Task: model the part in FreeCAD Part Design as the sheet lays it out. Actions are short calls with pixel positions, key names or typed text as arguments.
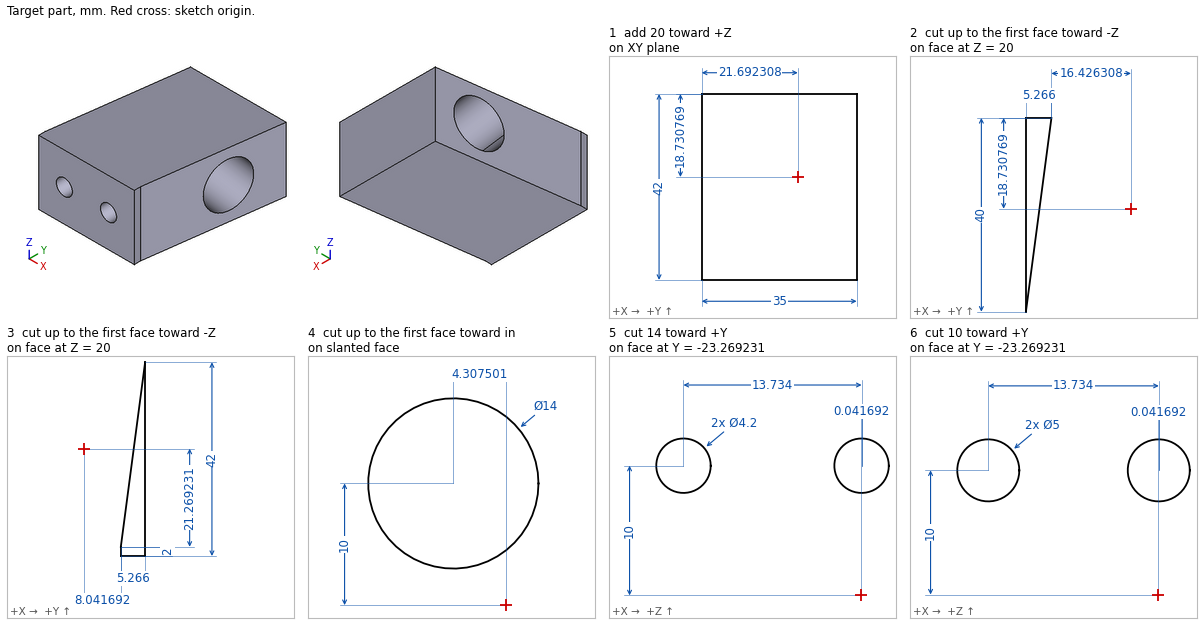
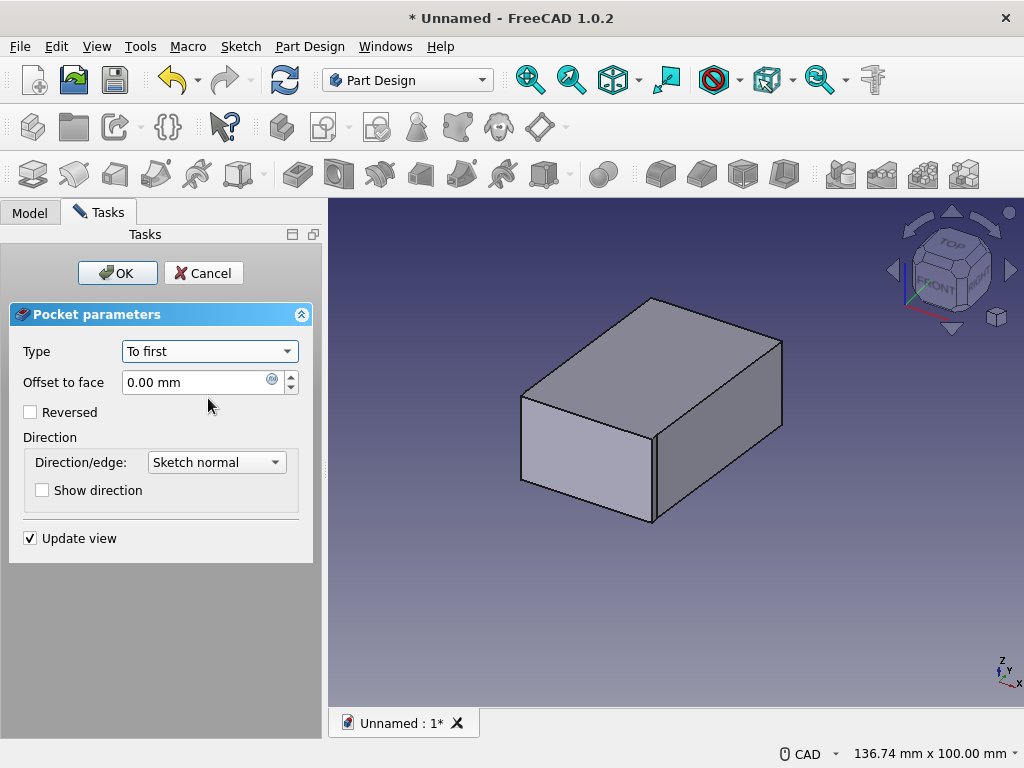
click(118, 273)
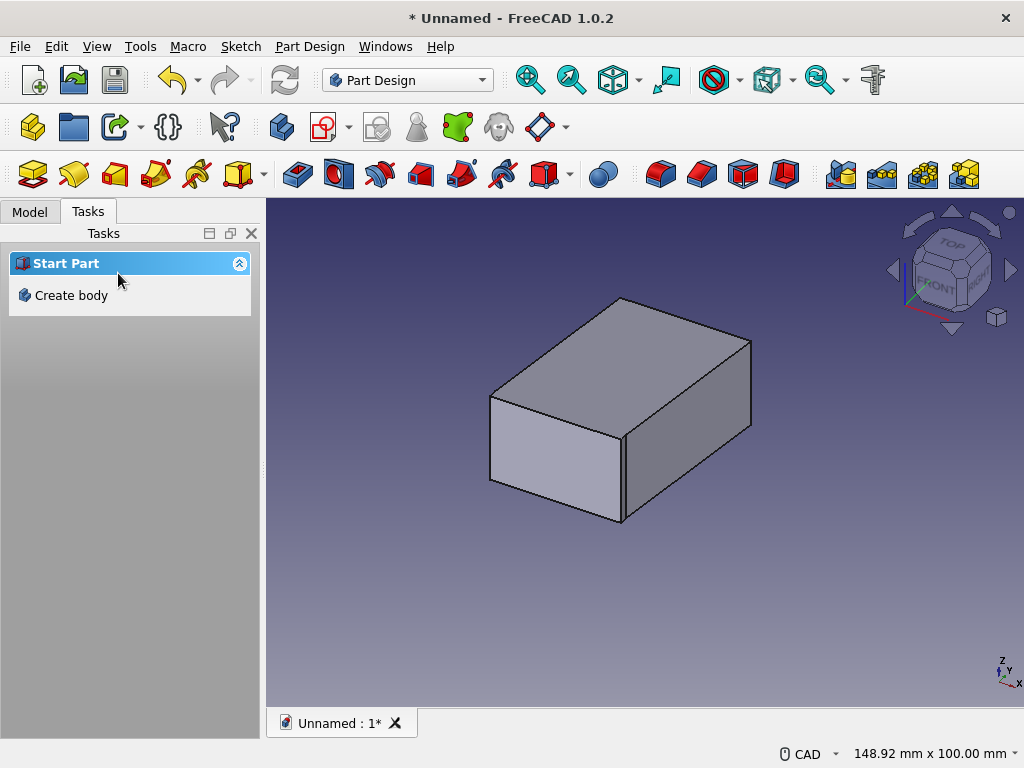
key(6)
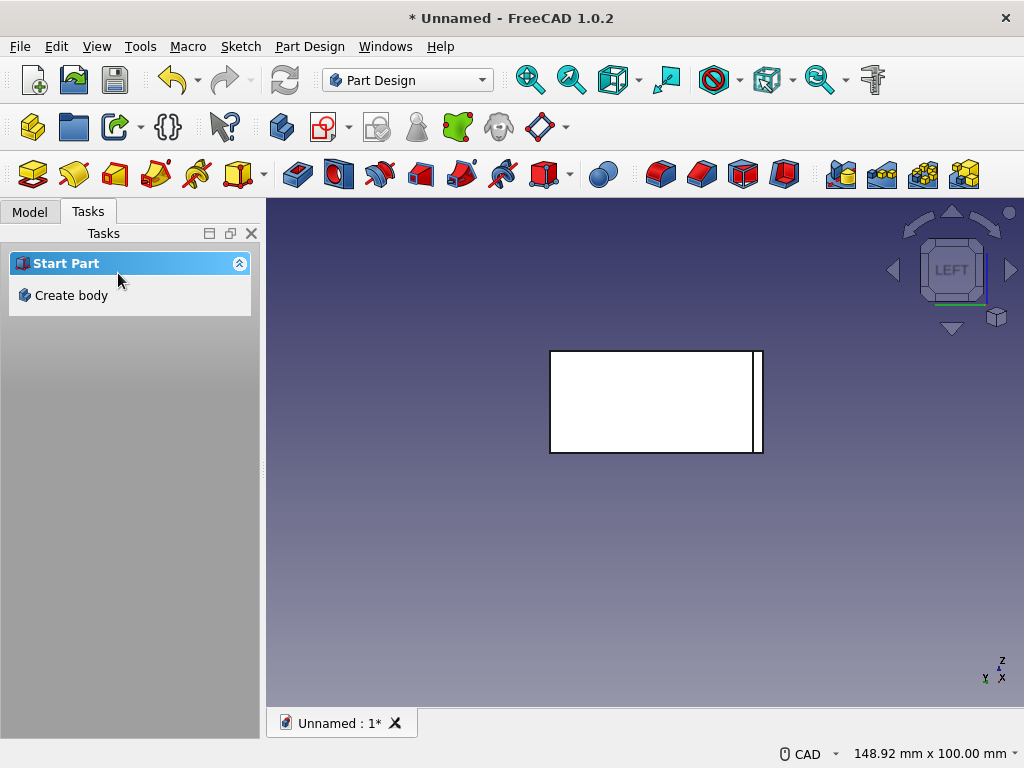
click(531, 80)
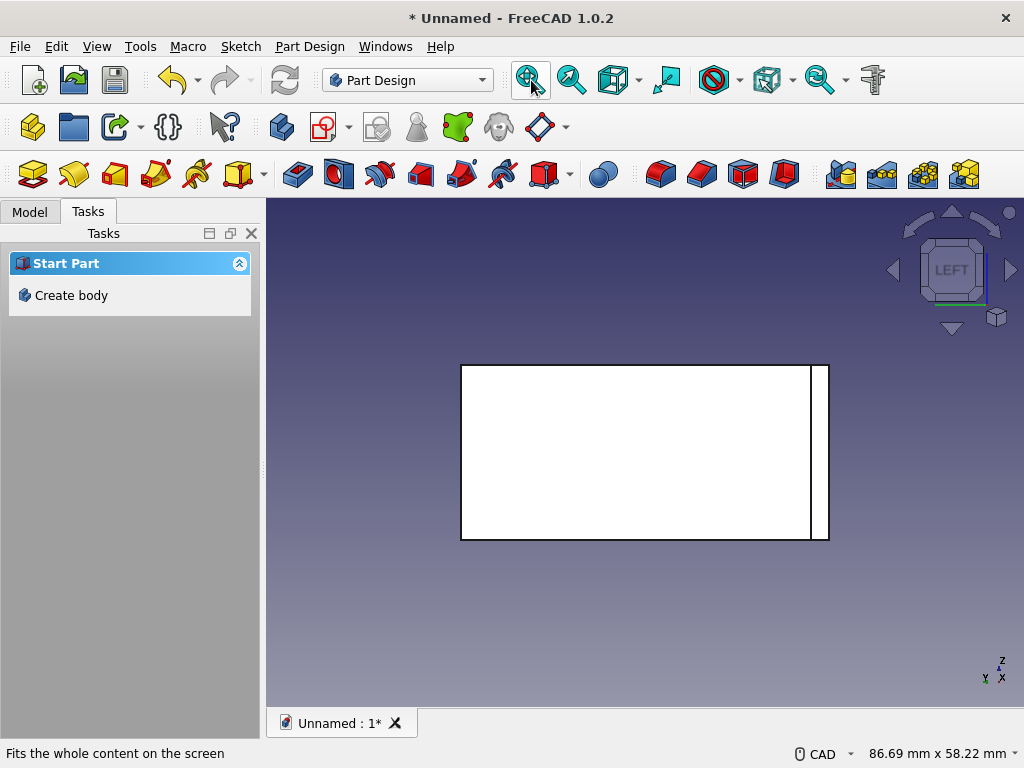
click(586, 451)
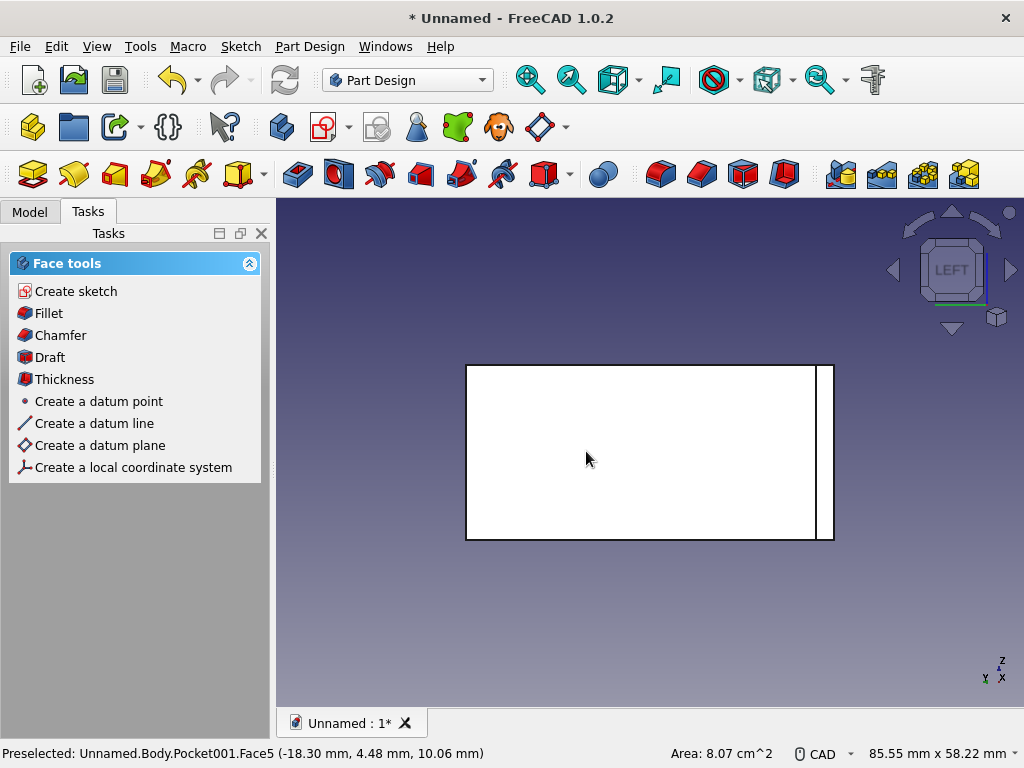
click(322, 128)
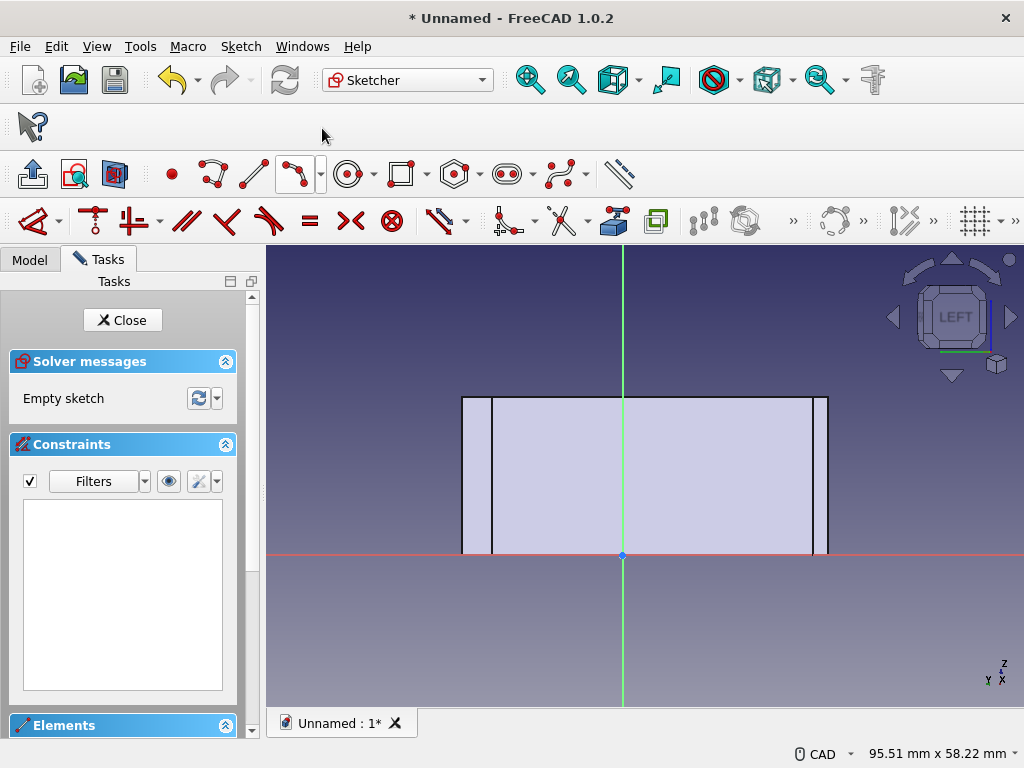
scroll(599, 498, up, 4)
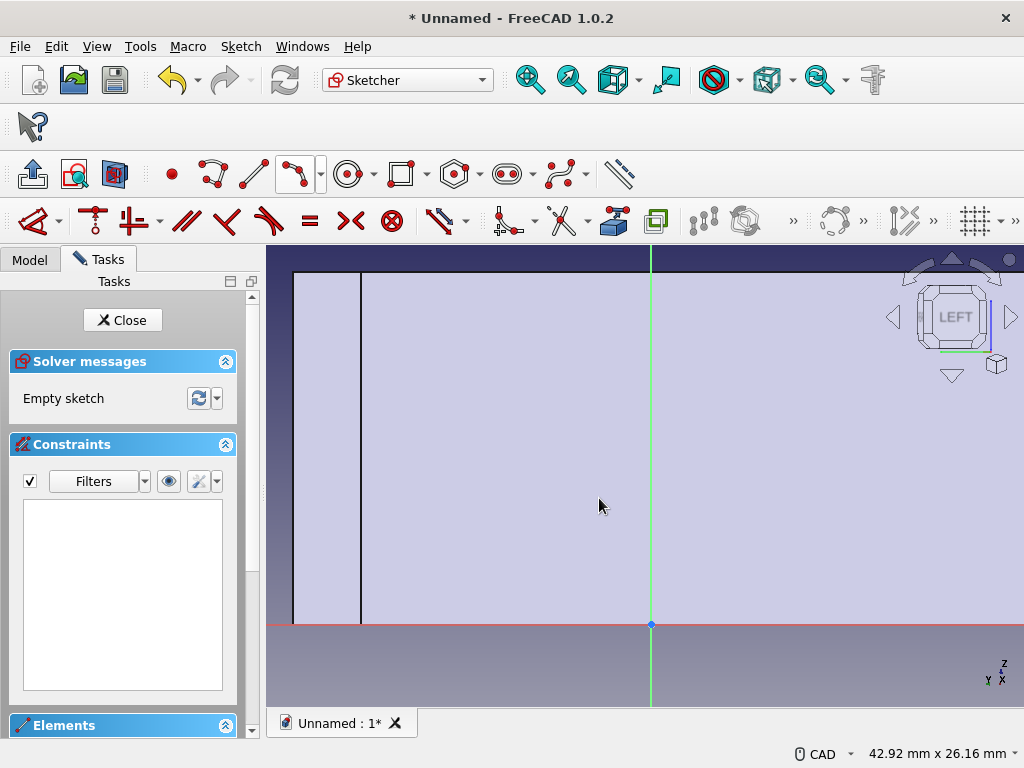
click(348, 174)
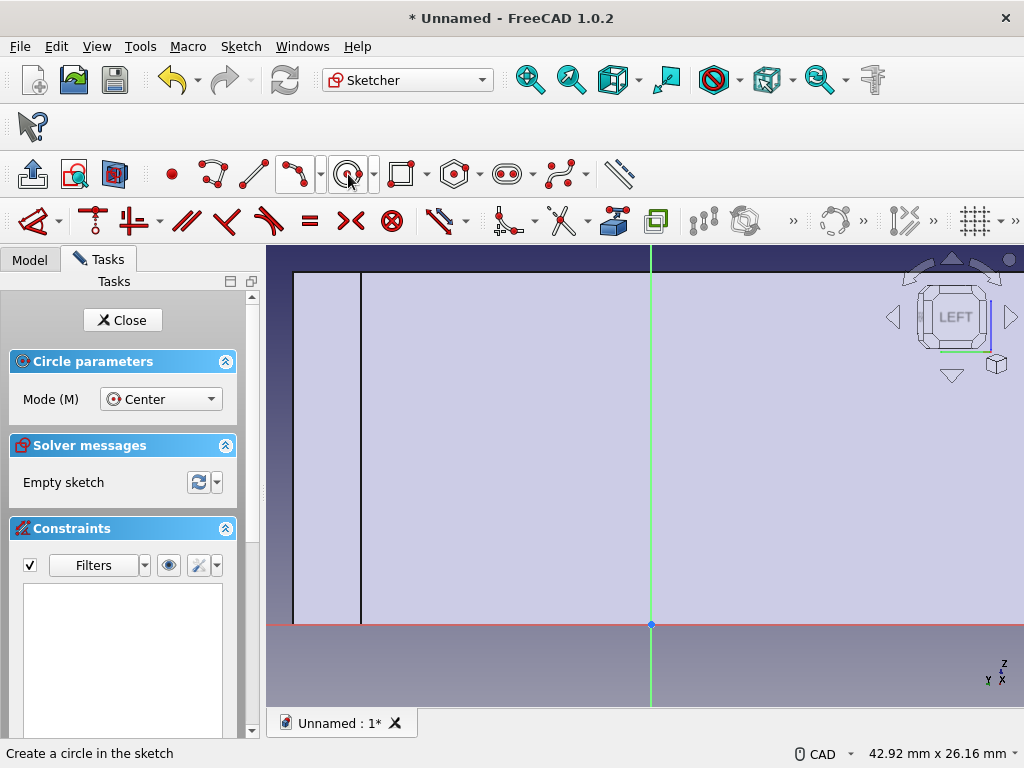
click(575, 448)
click(488, 361)
key(Escape)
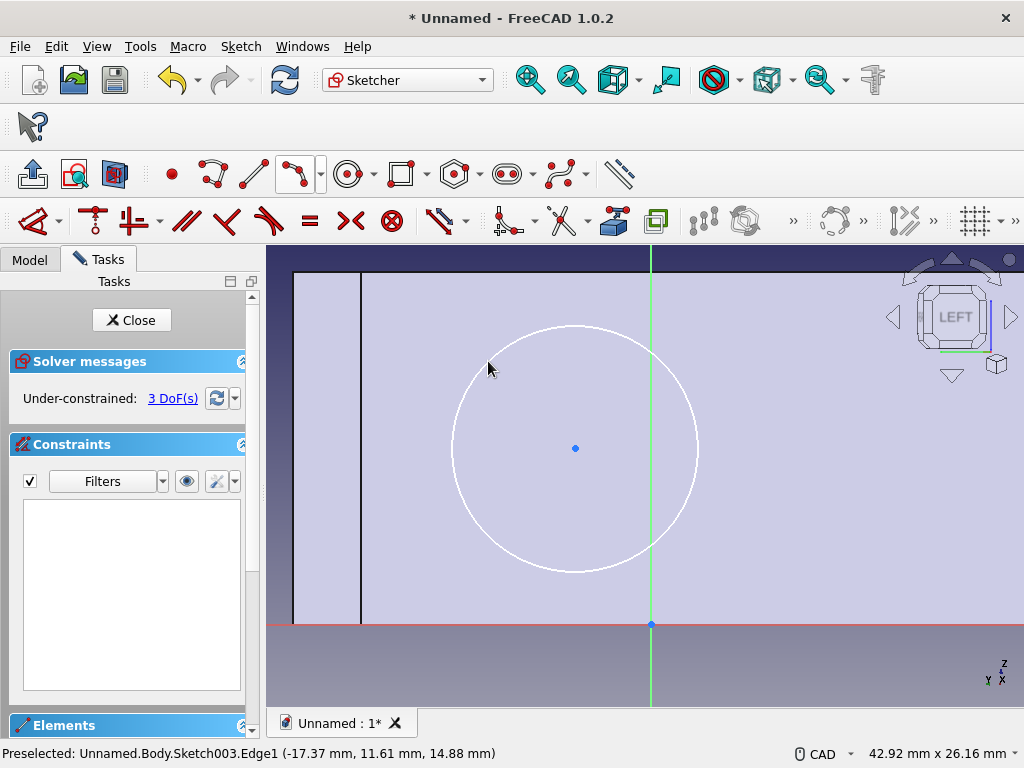
key(d)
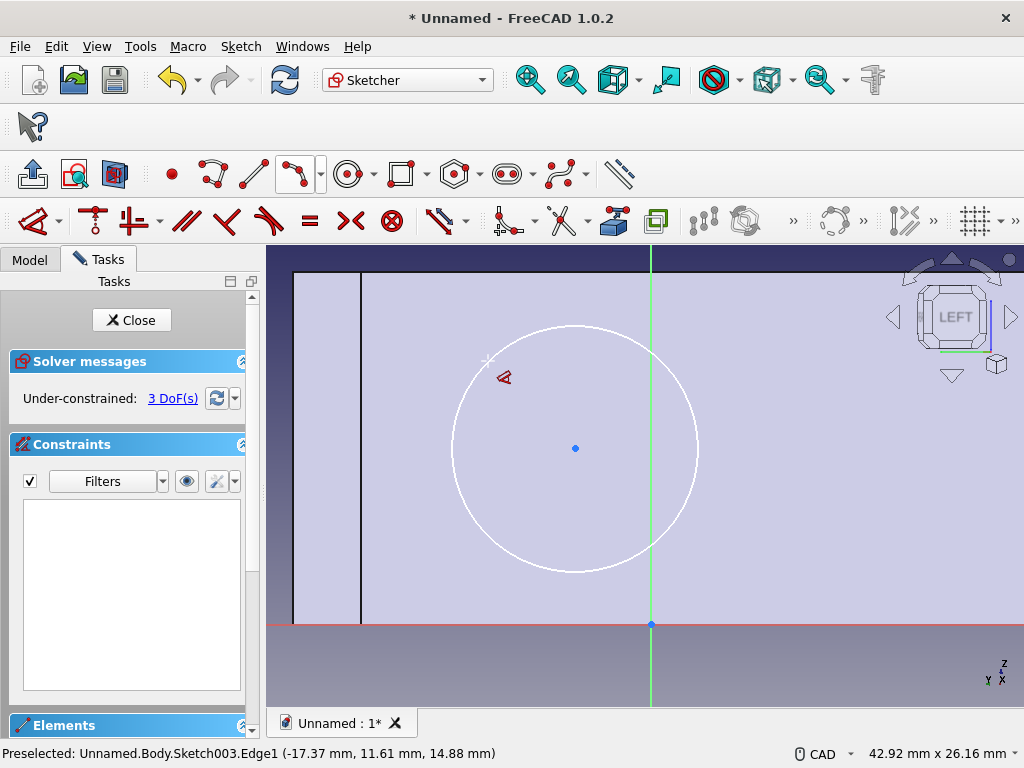
scroll(662, 362, up, 2)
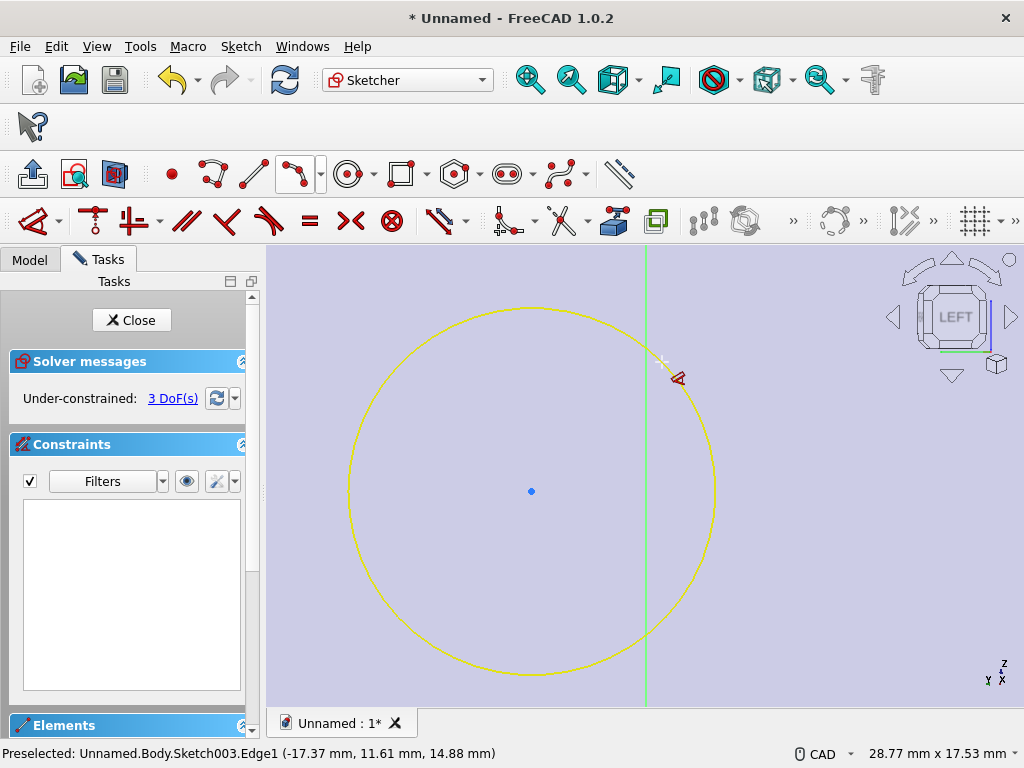
click(661, 361)
click(683, 338)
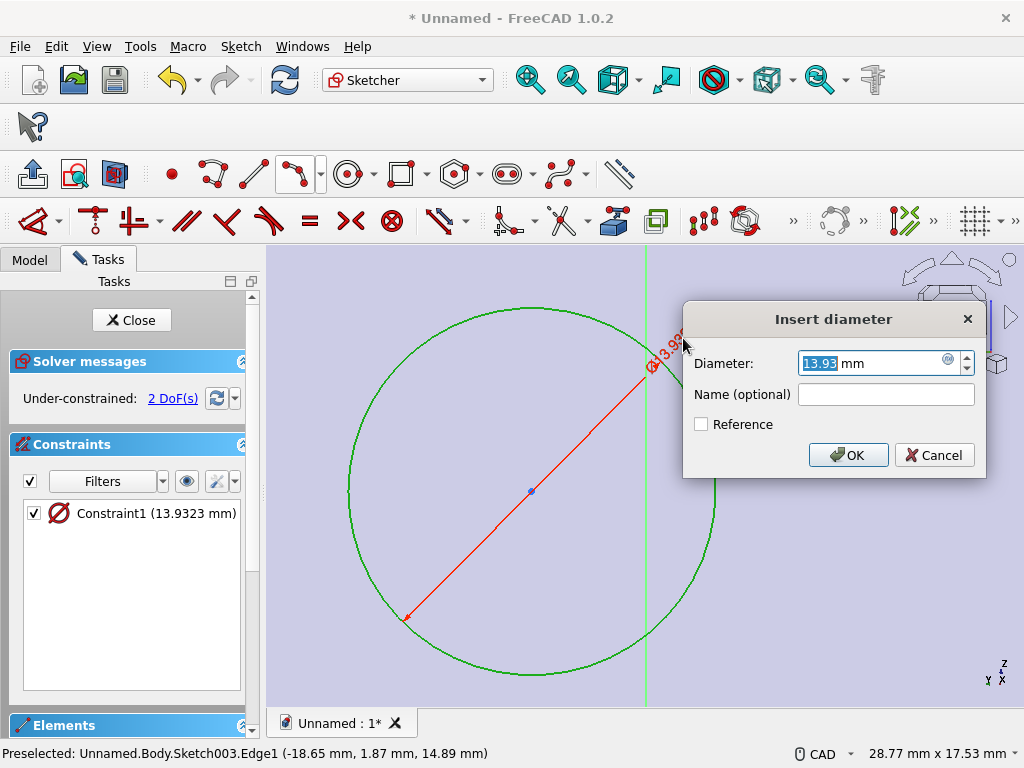
text(14)
key(Return)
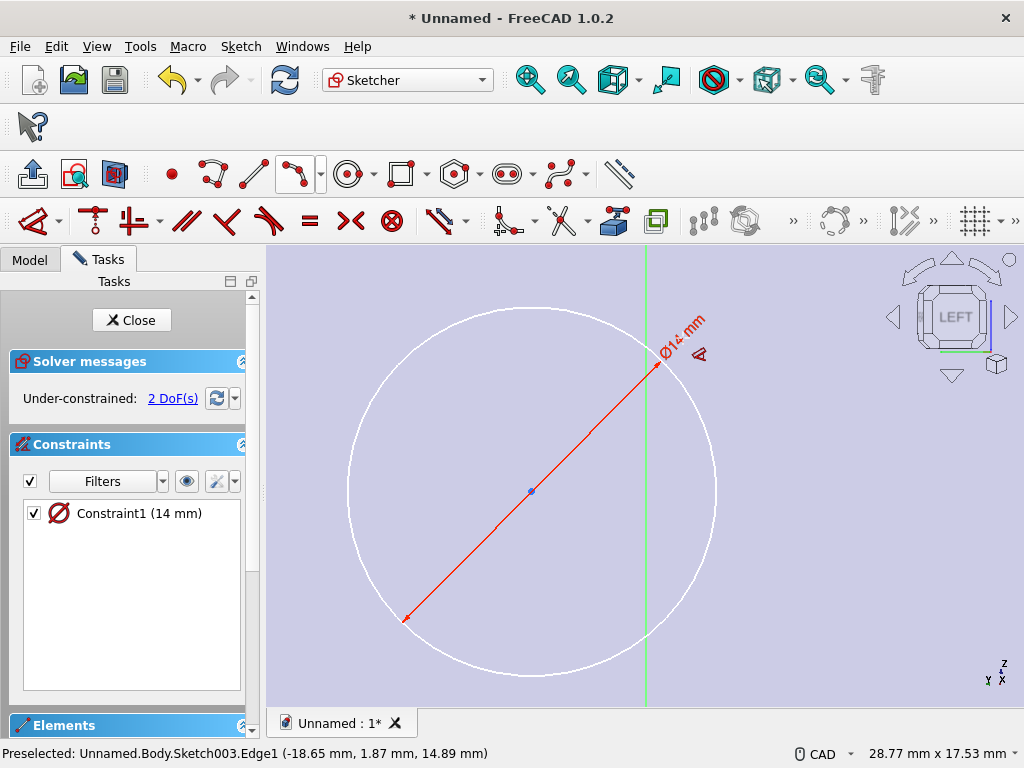
click(532, 492)
click(680, 542)